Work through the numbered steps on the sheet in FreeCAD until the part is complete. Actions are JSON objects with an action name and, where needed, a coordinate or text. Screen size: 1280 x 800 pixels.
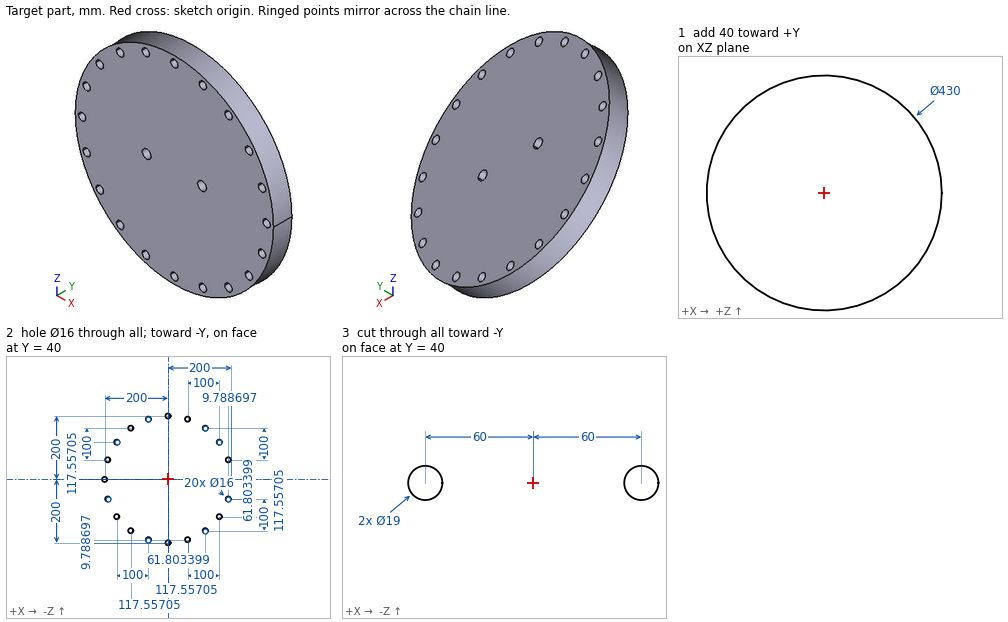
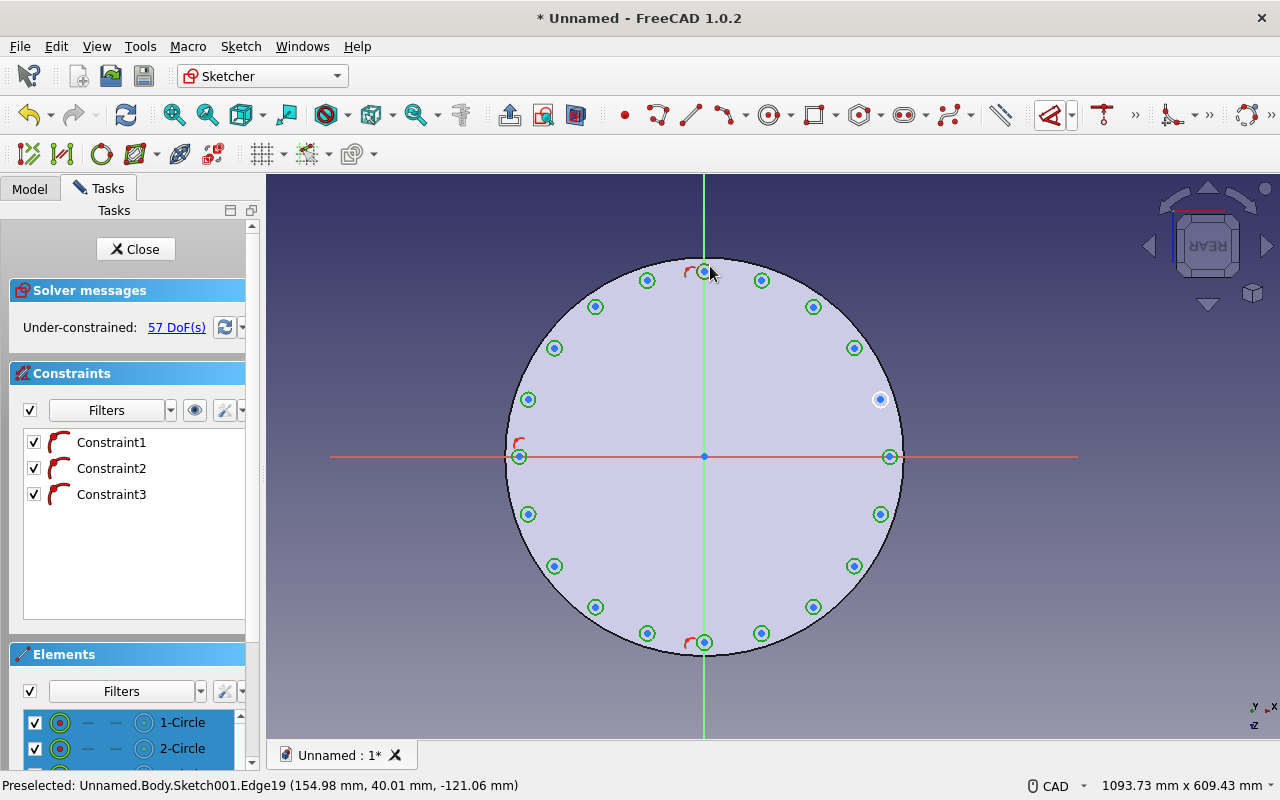
{"action": "scroll", "coordinate": [886, 394], "scroll_direction": "up", "scroll_amount": 3}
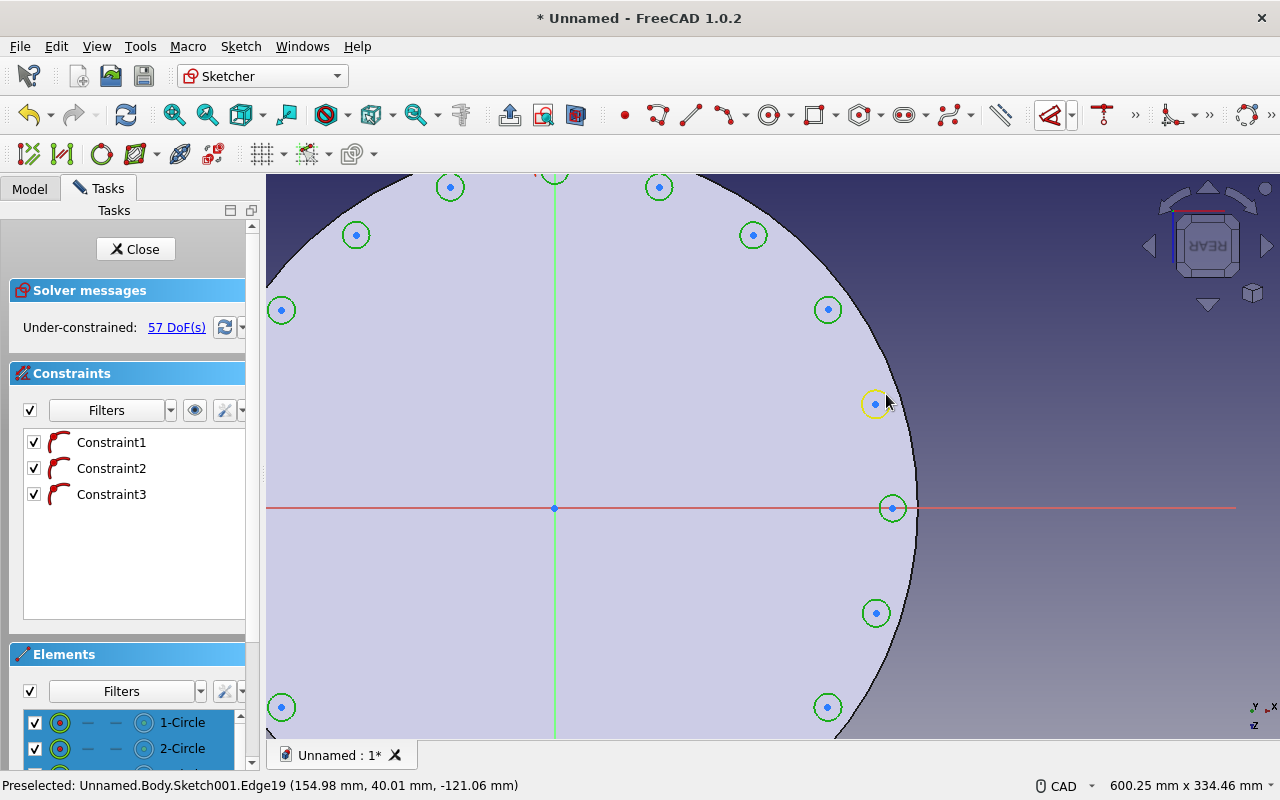
{"action": "left_click", "coordinate": [886, 394]}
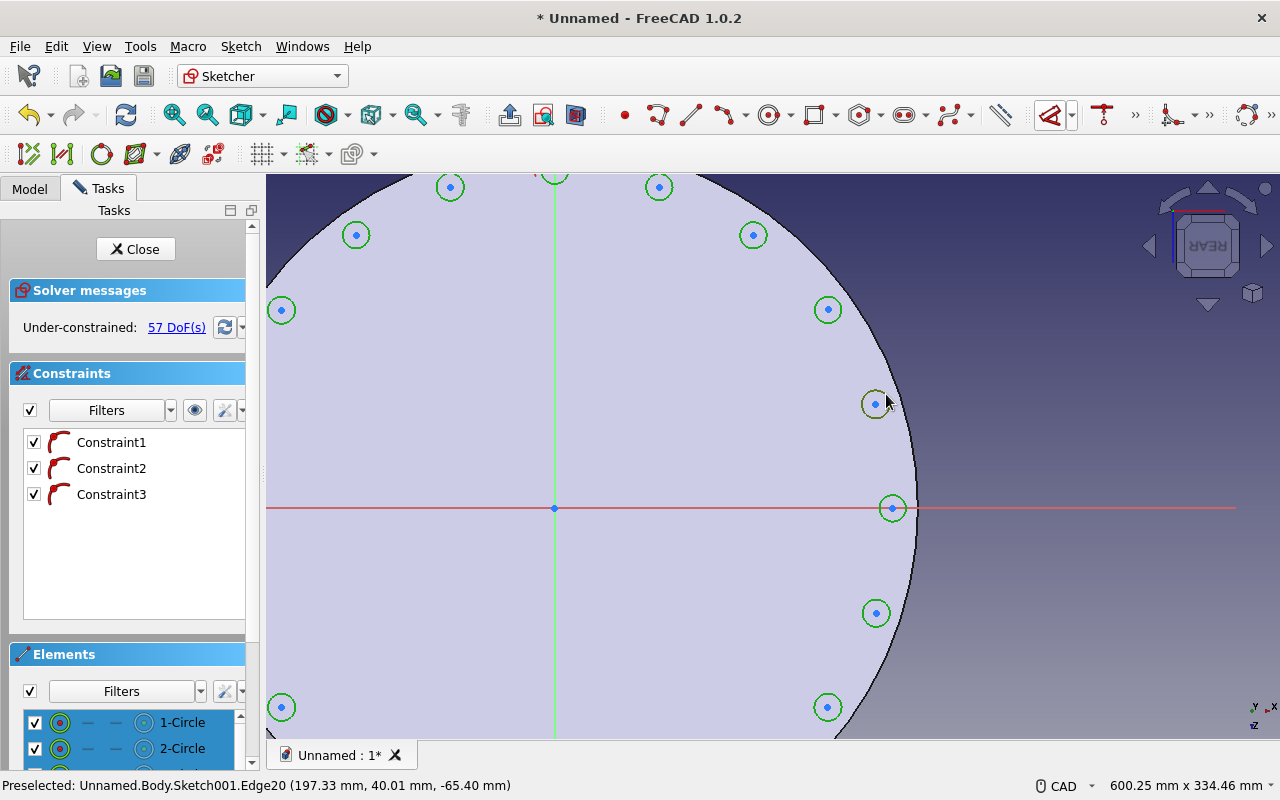
{"action": "key", "text": "e"}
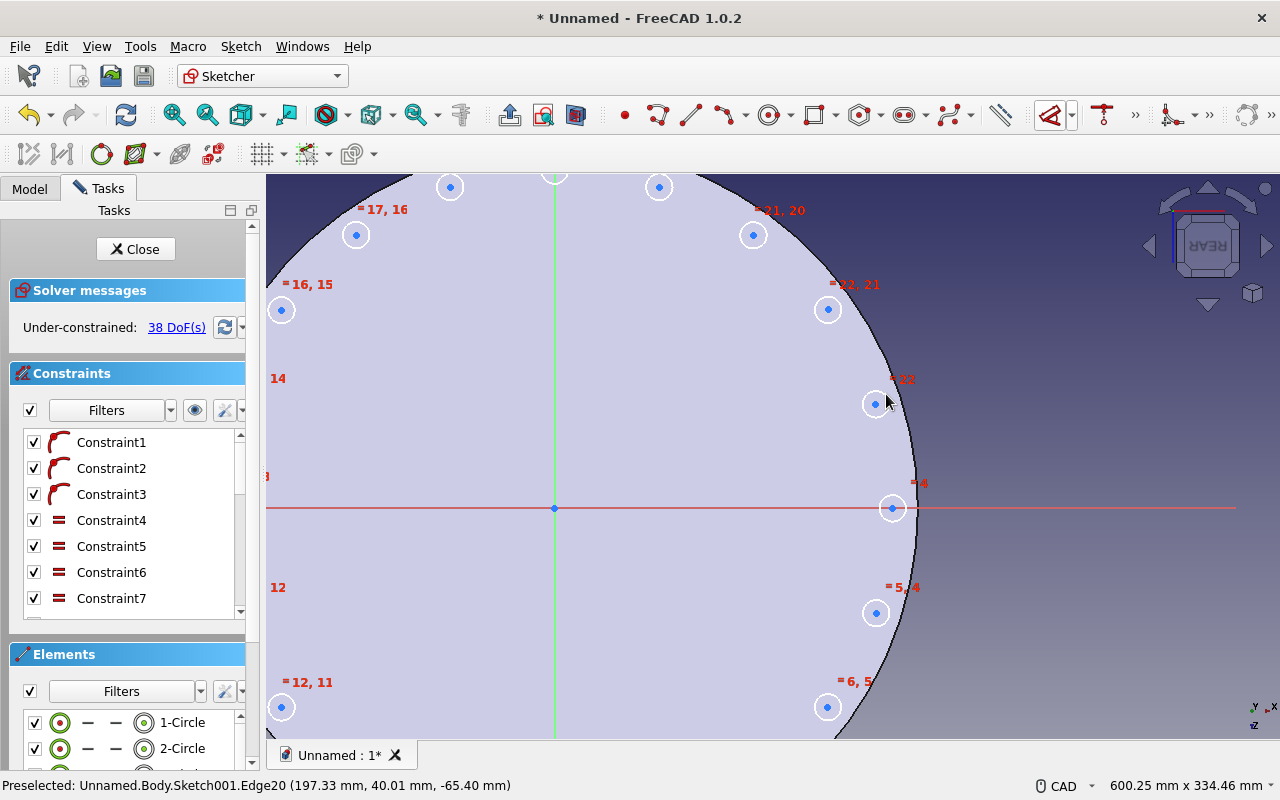
{"action": "left_click", "coordinate": [893, 508]}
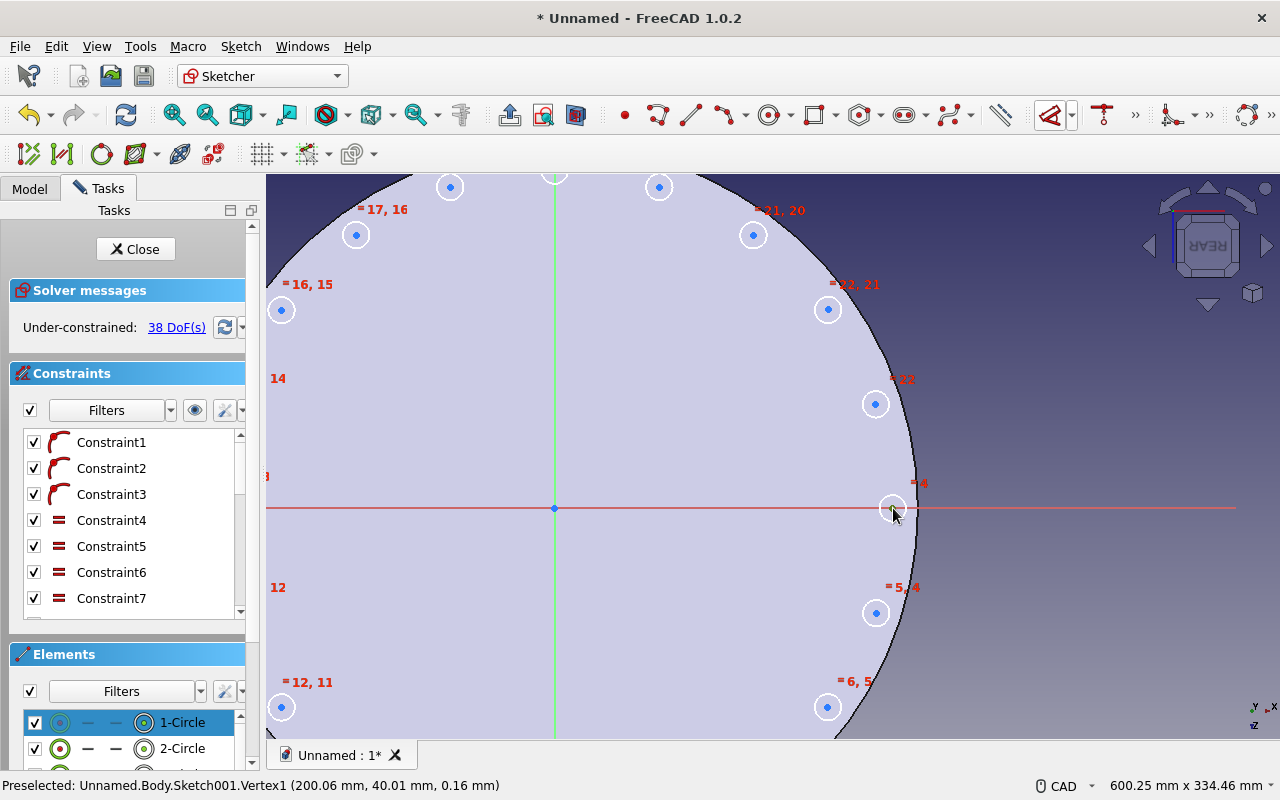
{"action": "left_click", "coordinate": [353, 508]}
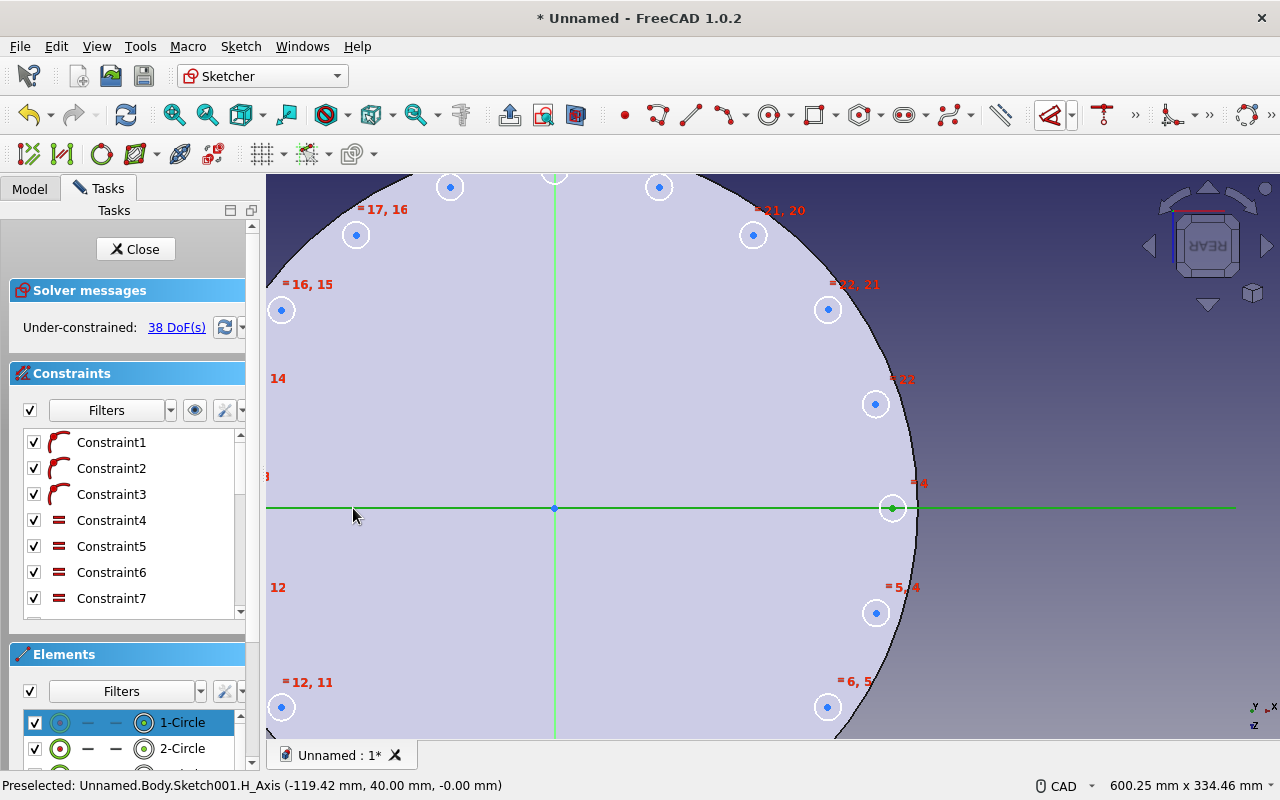
{"action": "key", "text": "c"}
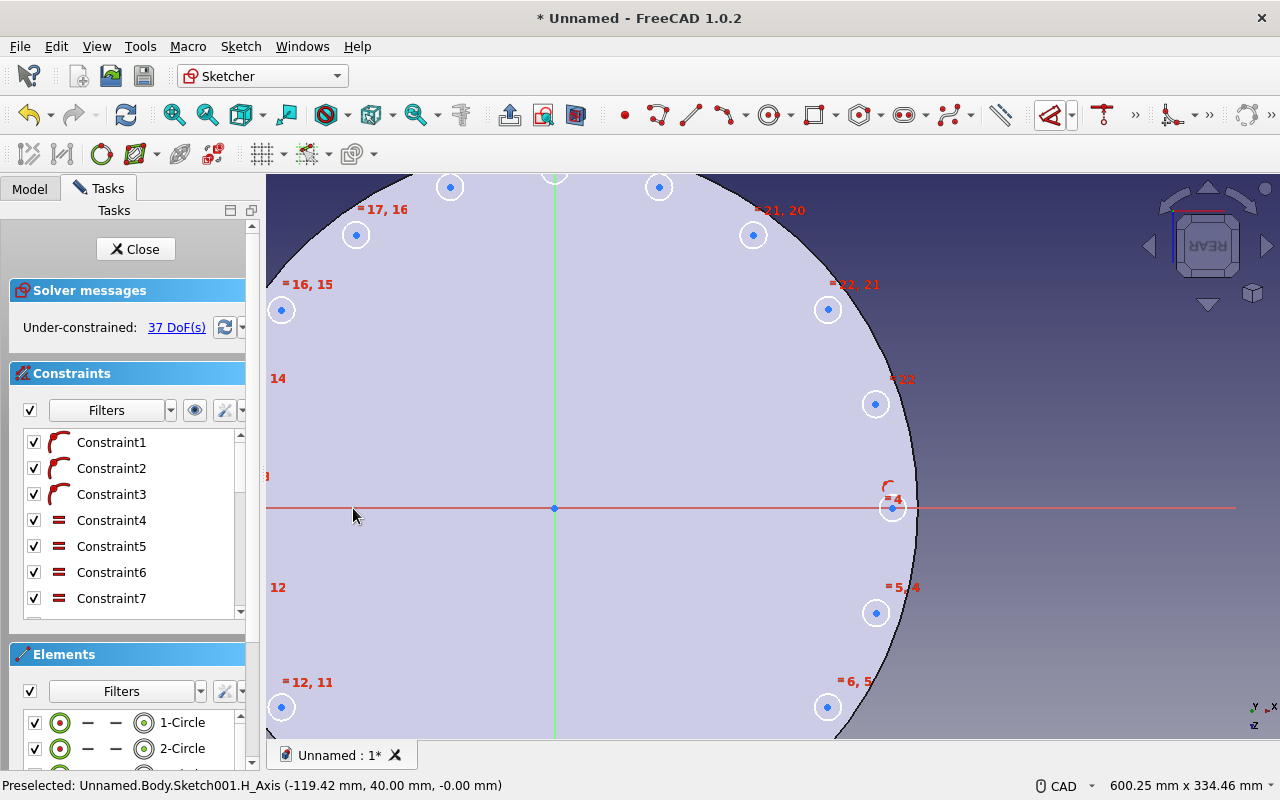
{"action": "scroll", "coordinate": [887, 394], "scroll_direction": "down", "scroll_amount": 3}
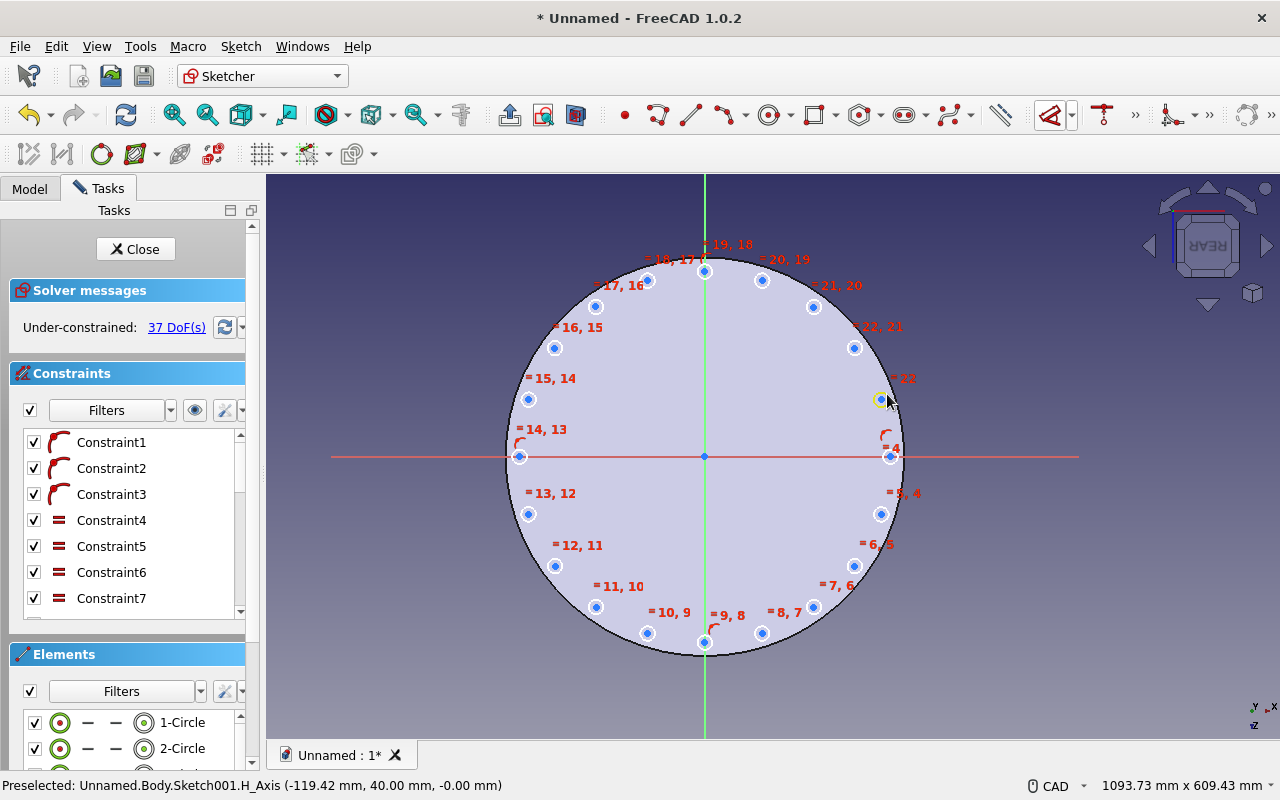
{"action": "left_click", "coordinate": [762, 634]}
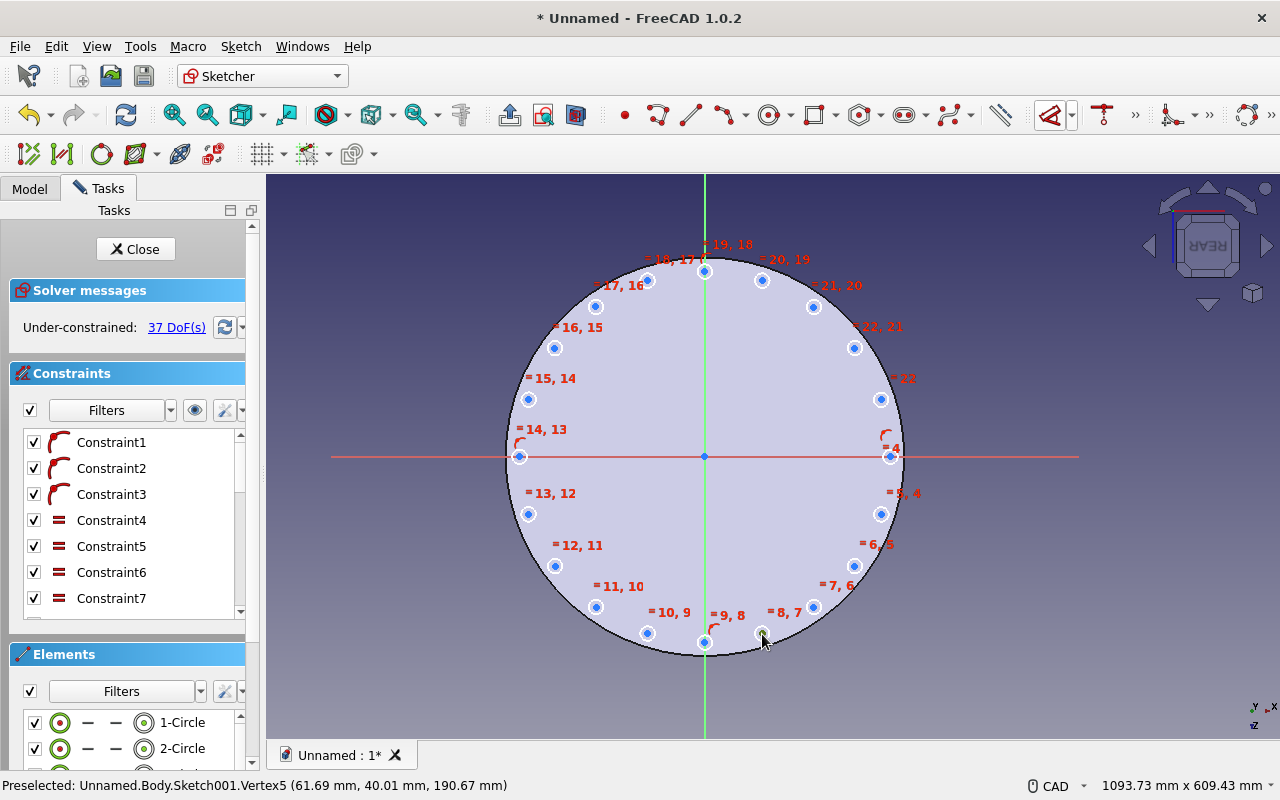
{"action": "left_click", "coordinate": [648, 634]}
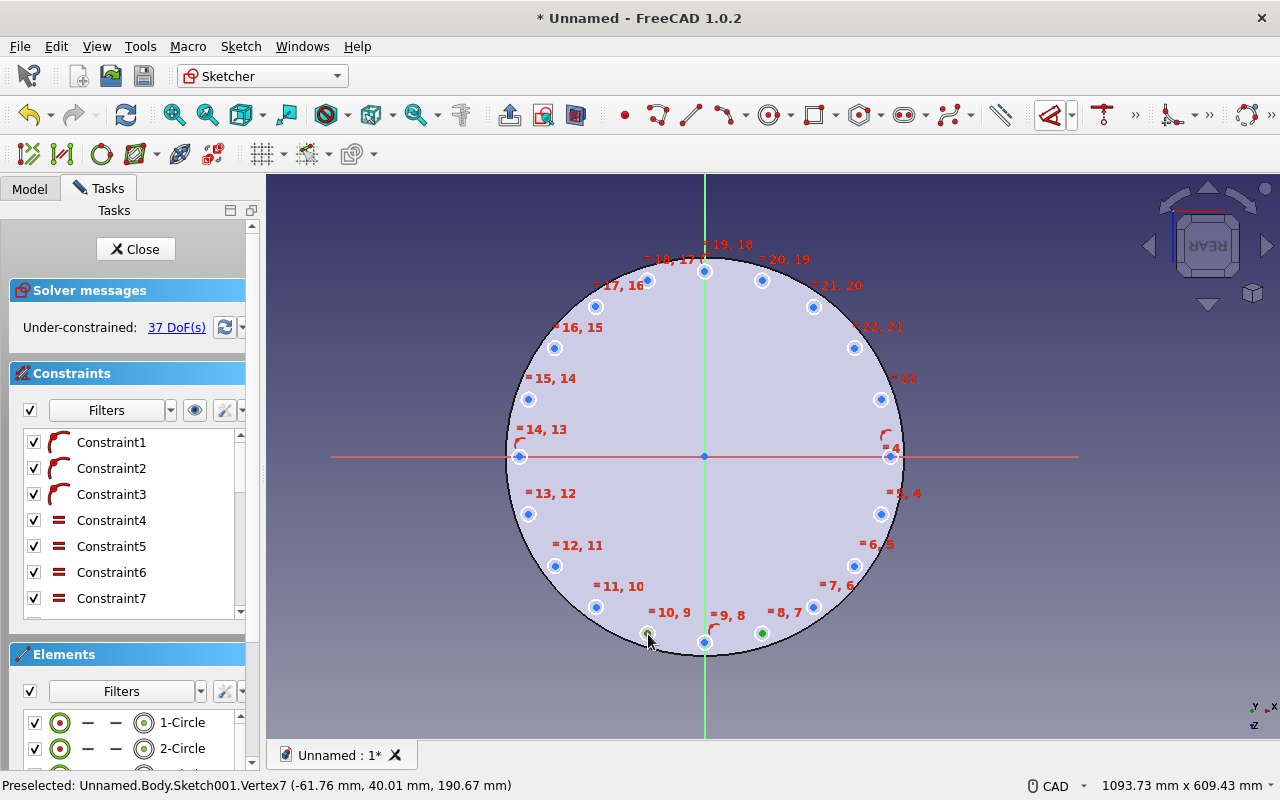
{"action": "key", "text": "h"}